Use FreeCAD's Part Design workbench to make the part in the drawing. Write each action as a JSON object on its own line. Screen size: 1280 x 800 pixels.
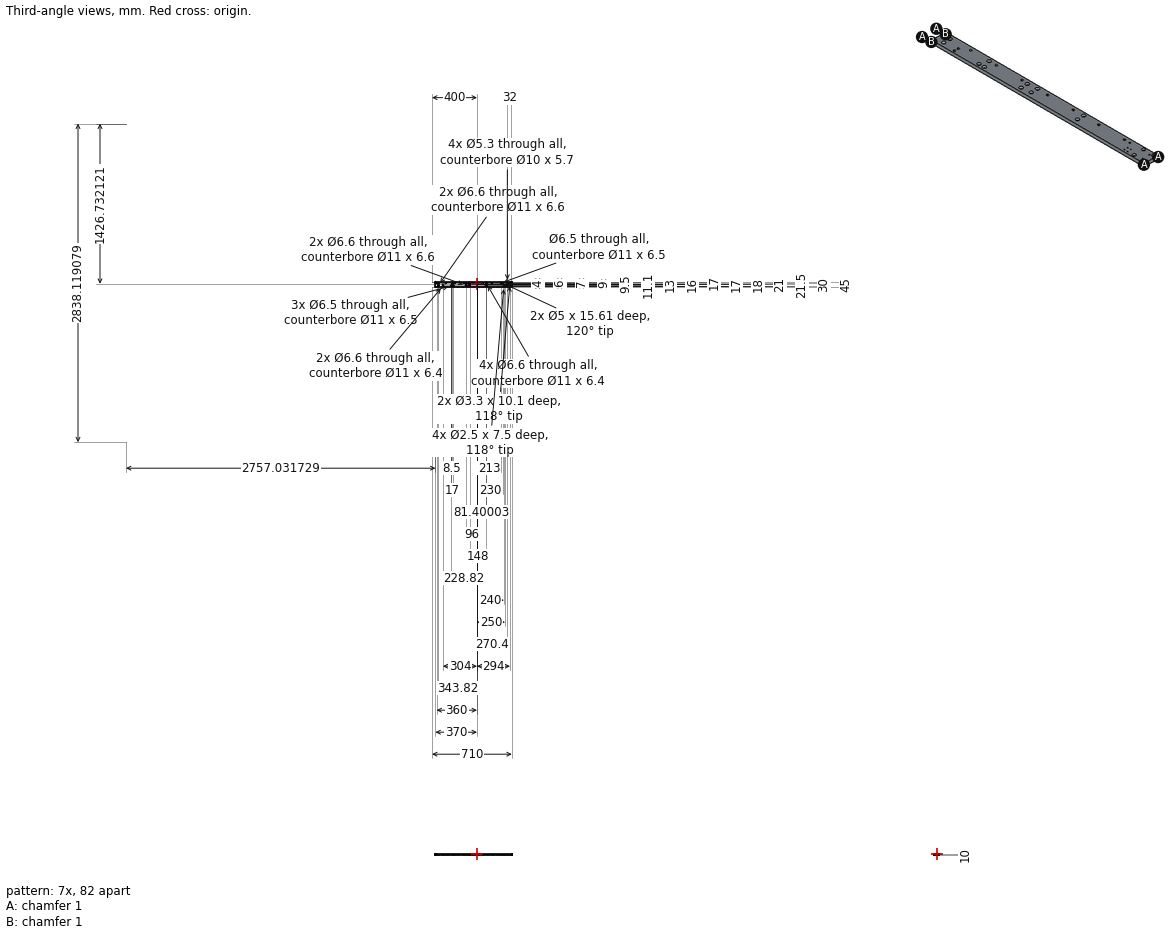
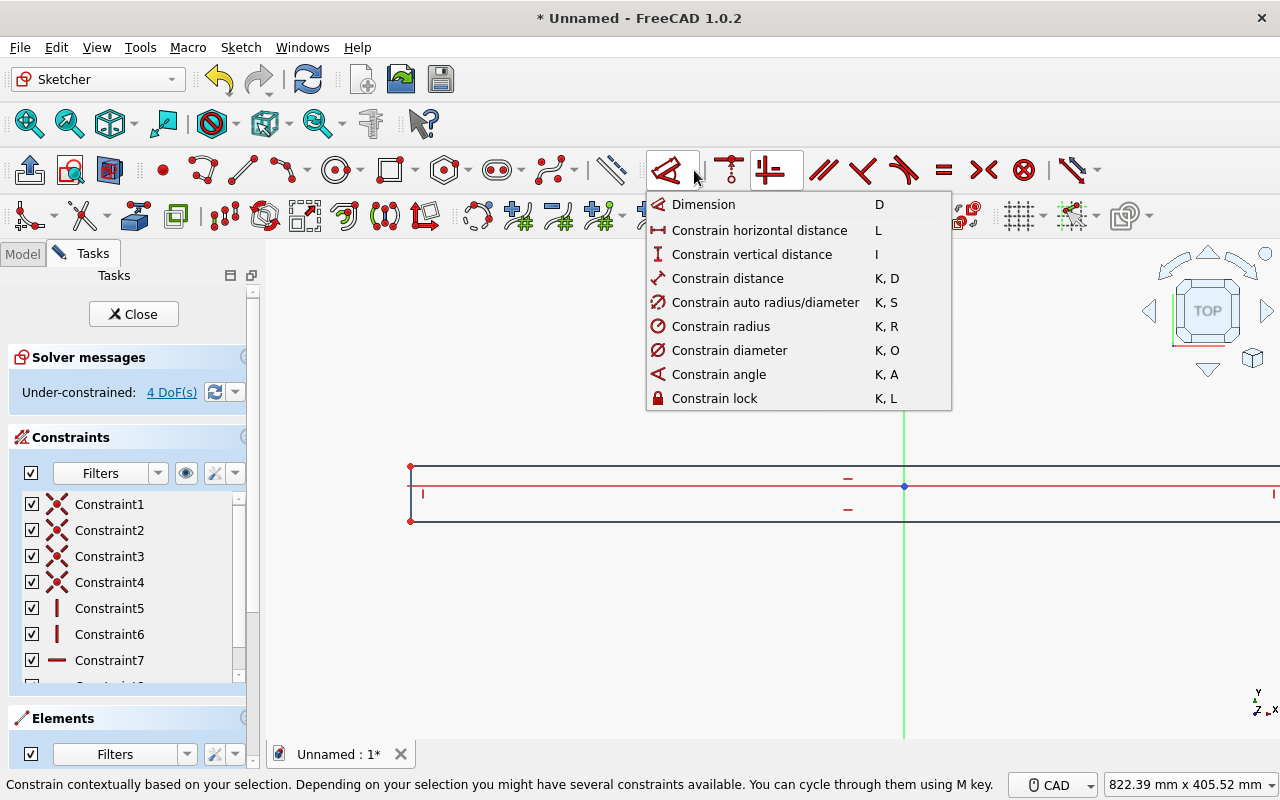
{"action": "left_click", "coordinate": [799, 254]}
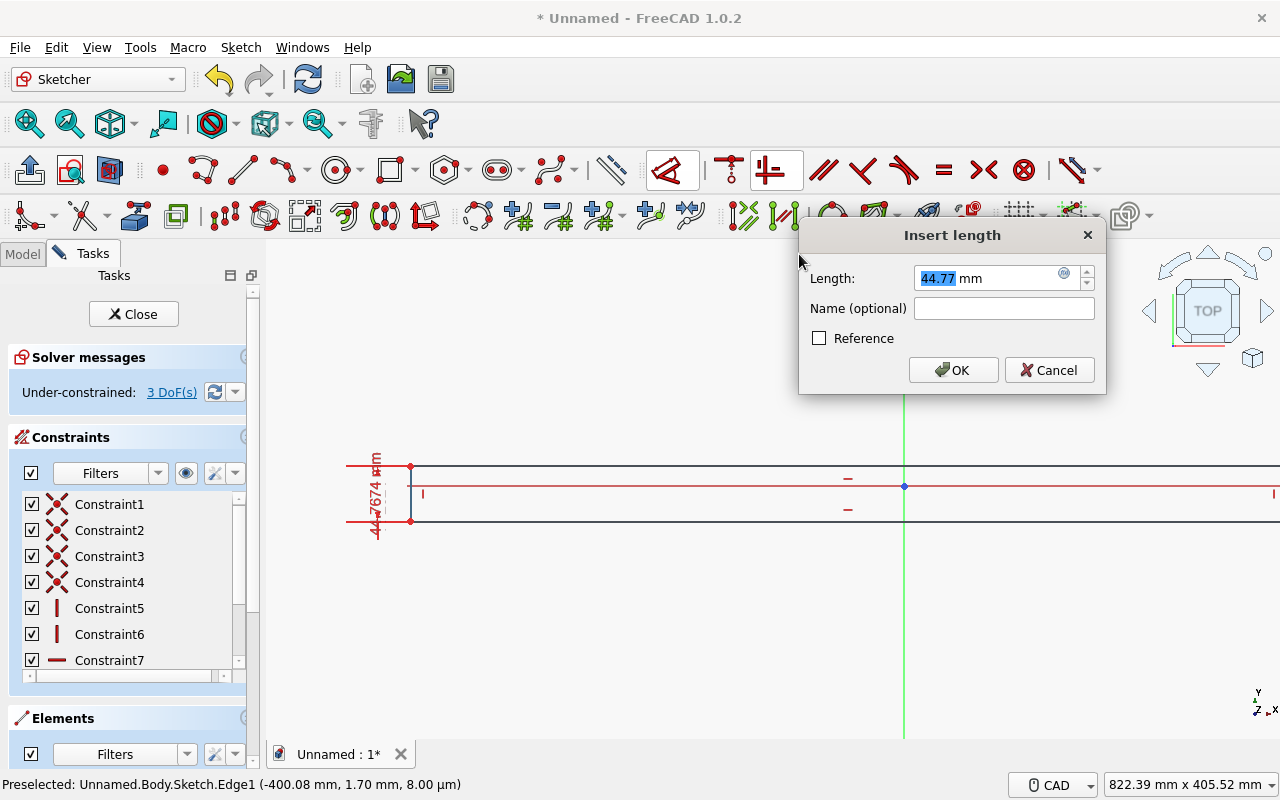
{"action": "type", "text": "45"}
{"action": "key", "text": "Return"}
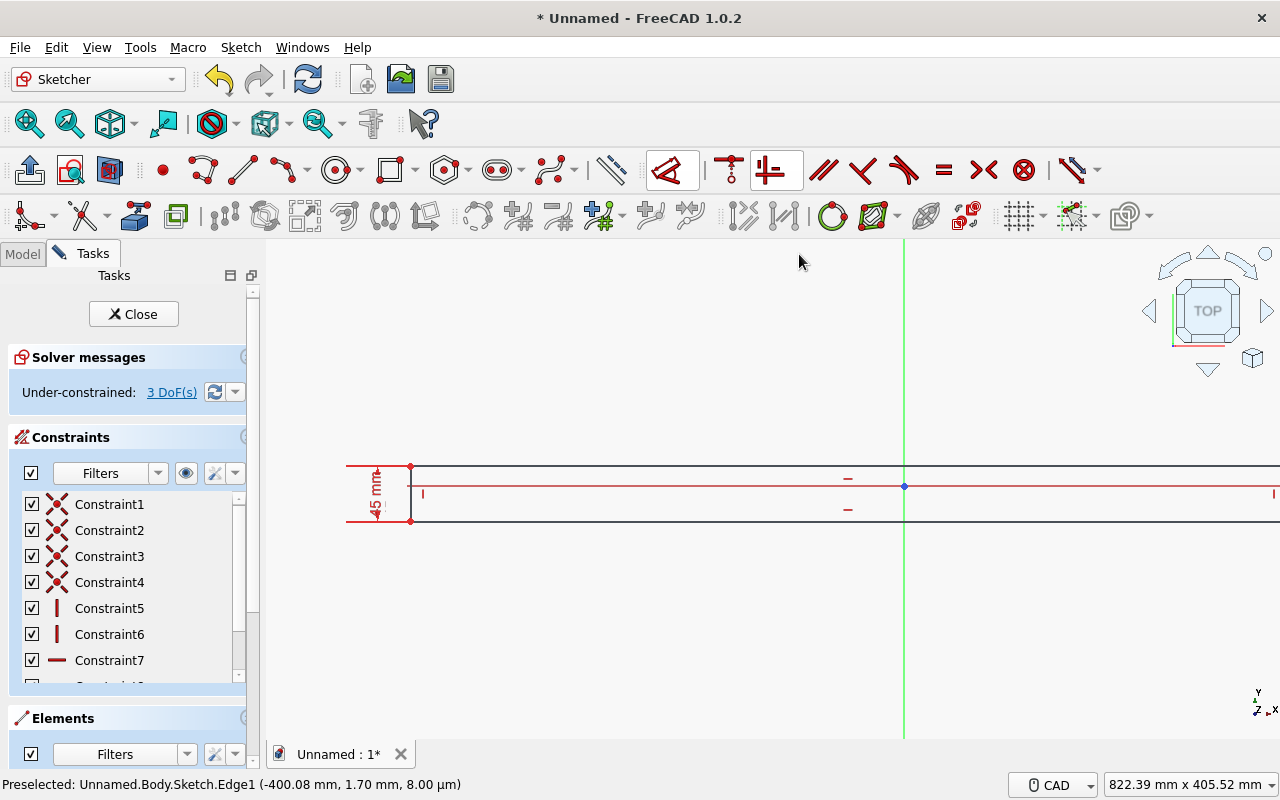
{"action": "left_click", "coordinate": [674, 522]}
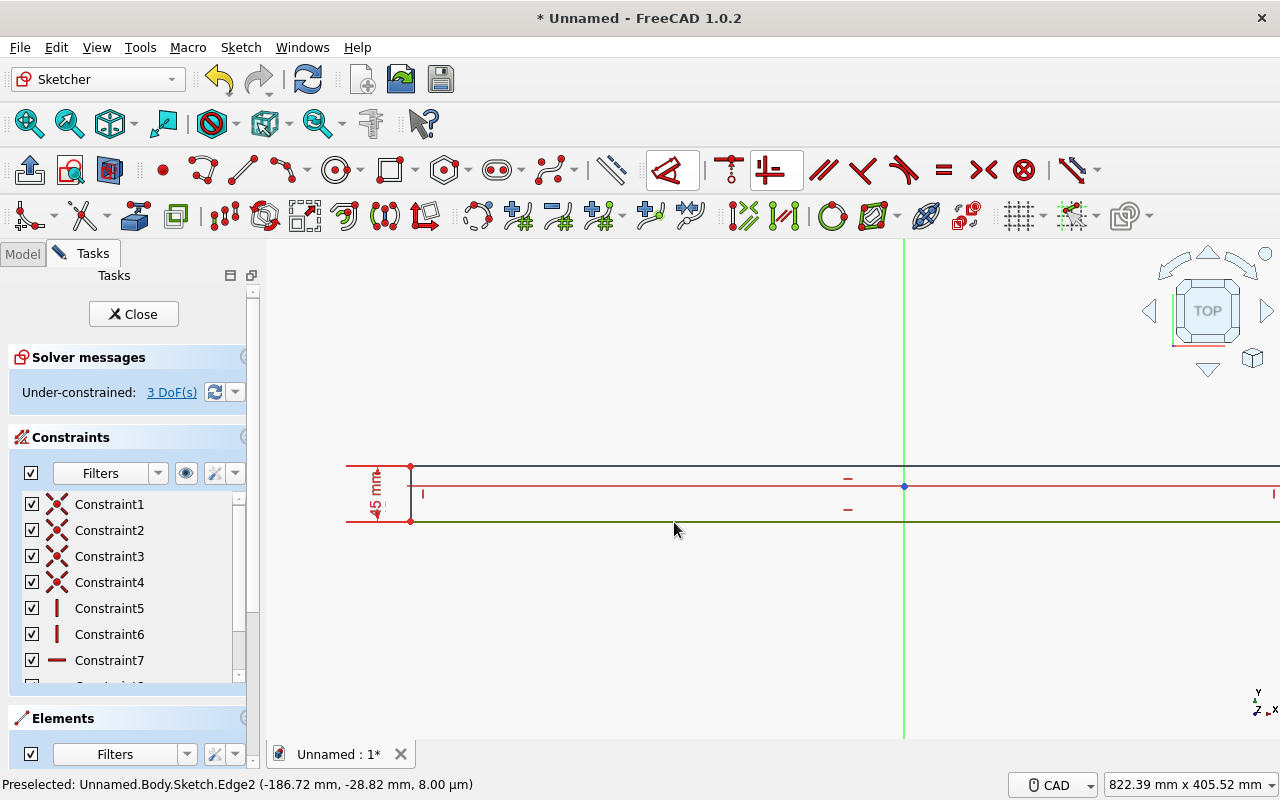
{"action": "key", "text": "l"}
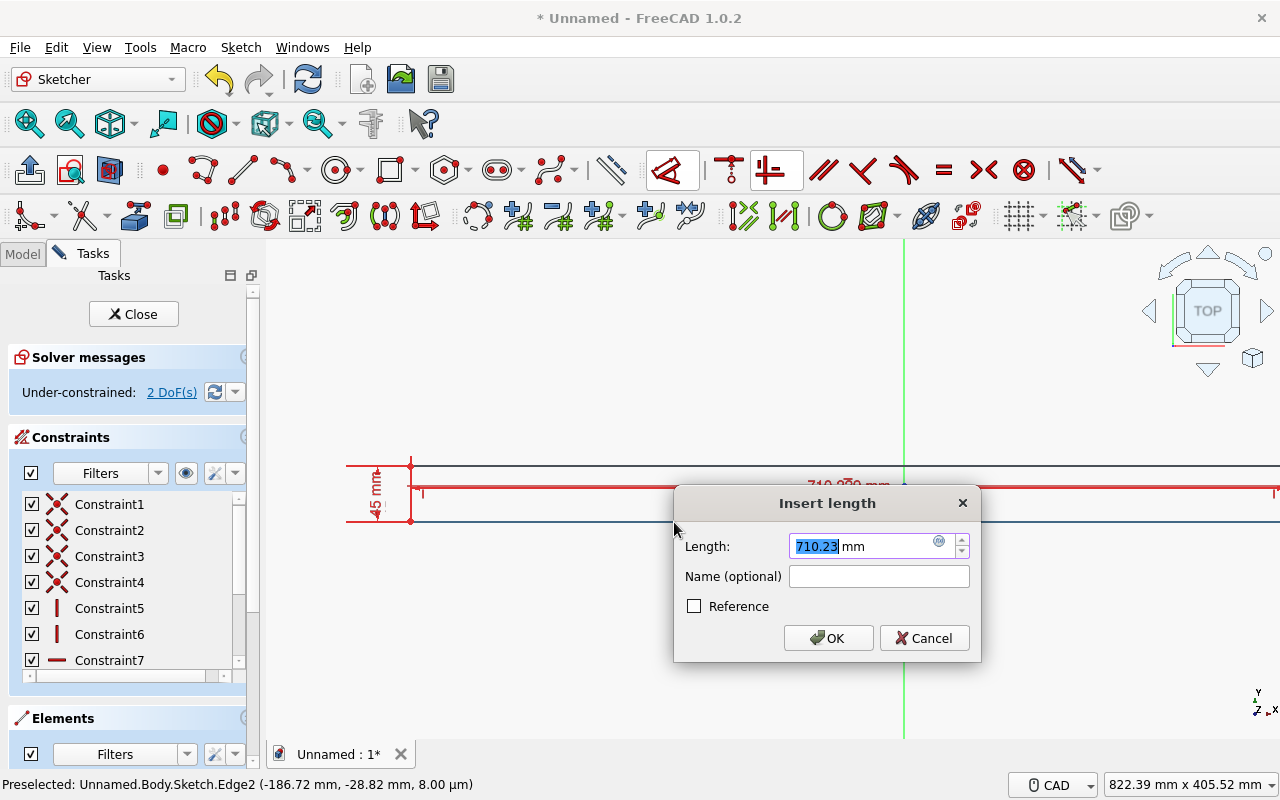
{"action": "type", "text": "710"}
{"action": "key", "text": "Return"}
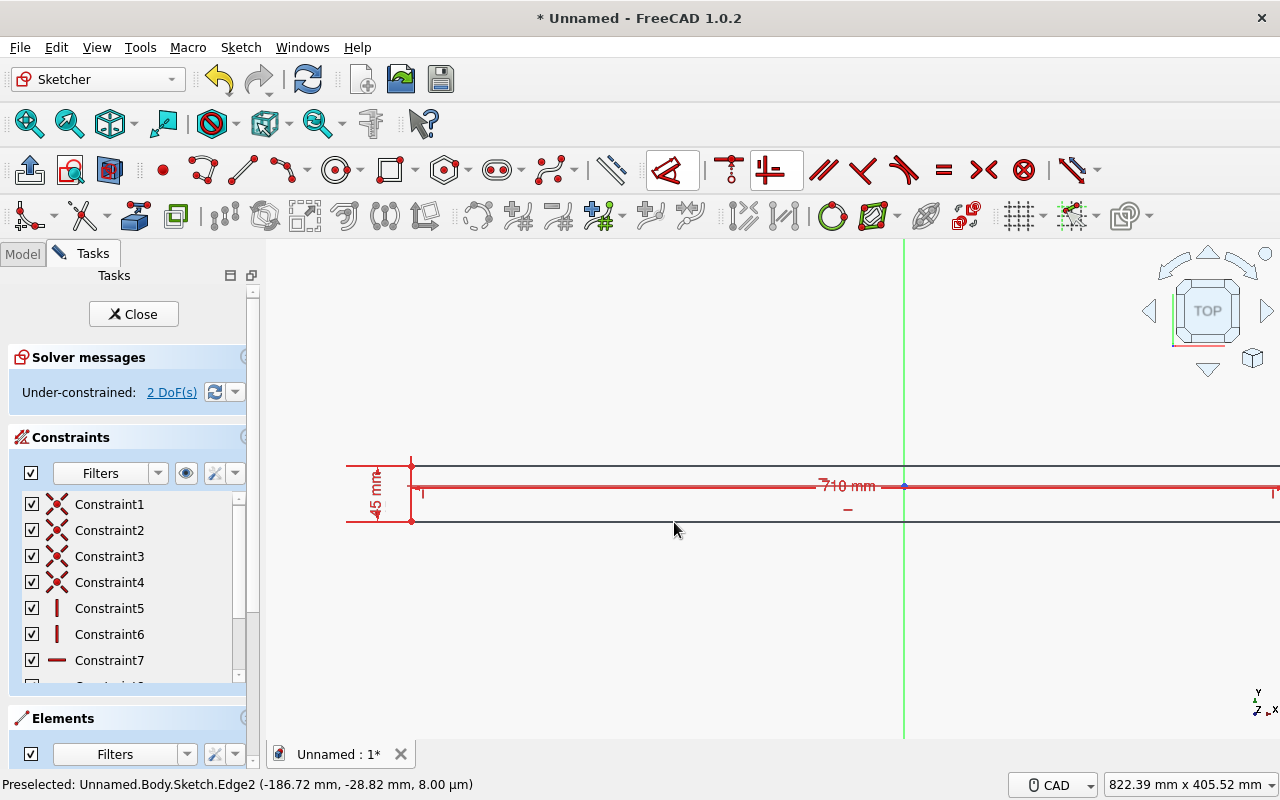
{"action": "scroll", "coordinate": [411, 466], "scroll_direction": "up", "scroll_amount": 4}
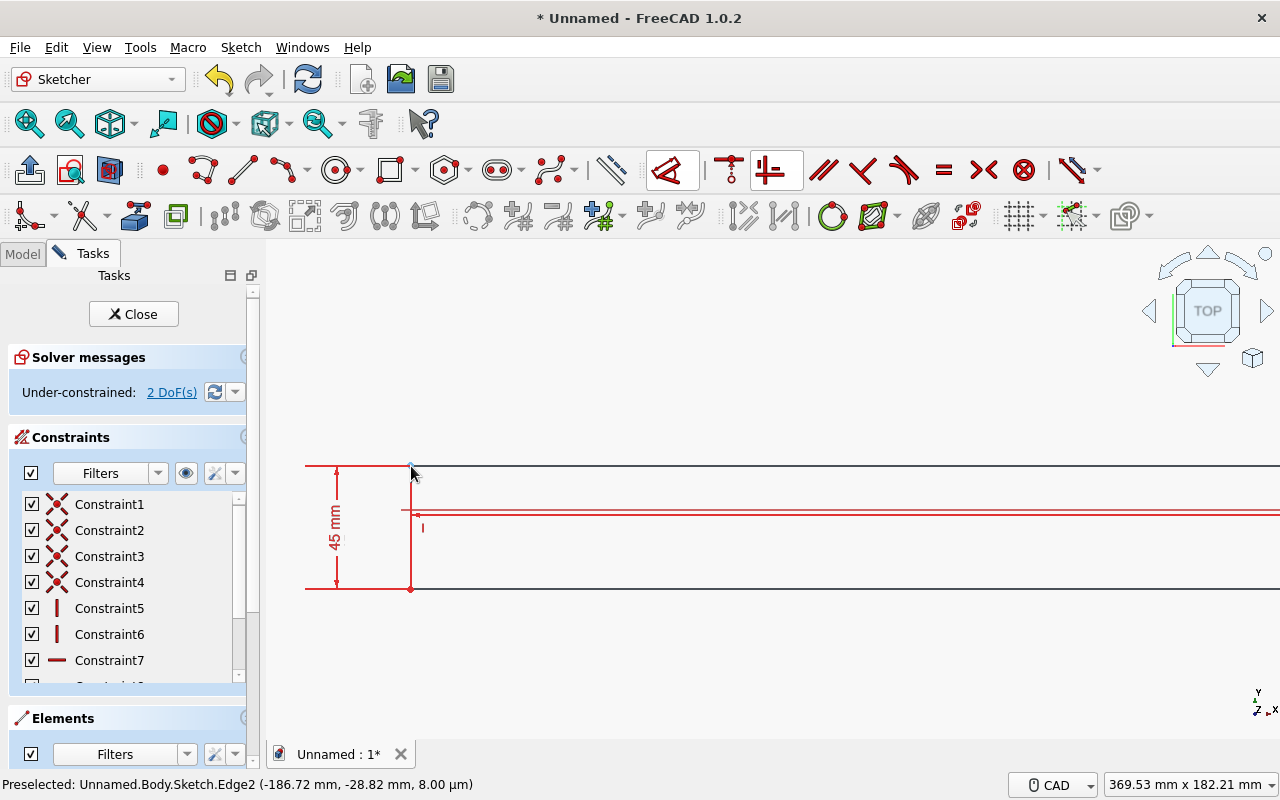
{"action": "left_click", "coordinate": [411, 466]}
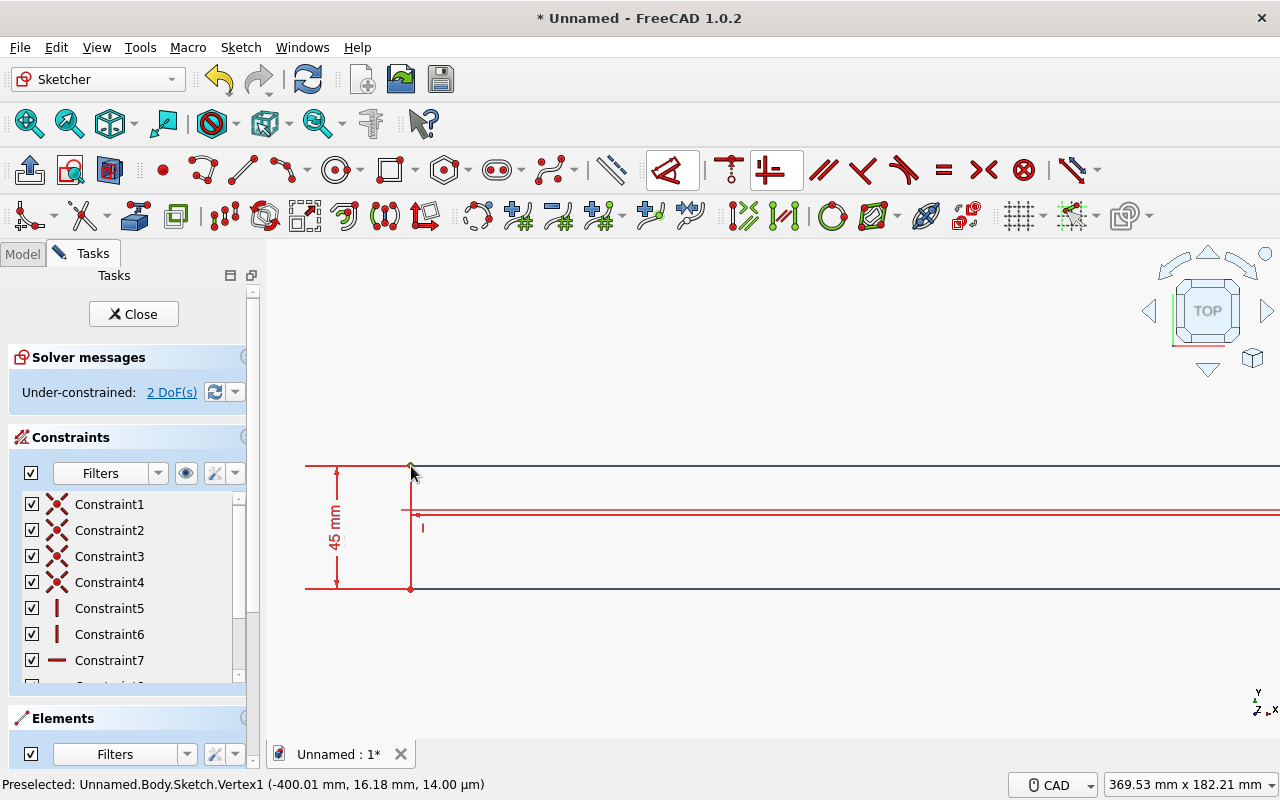
{"action": "key", "text": "i"}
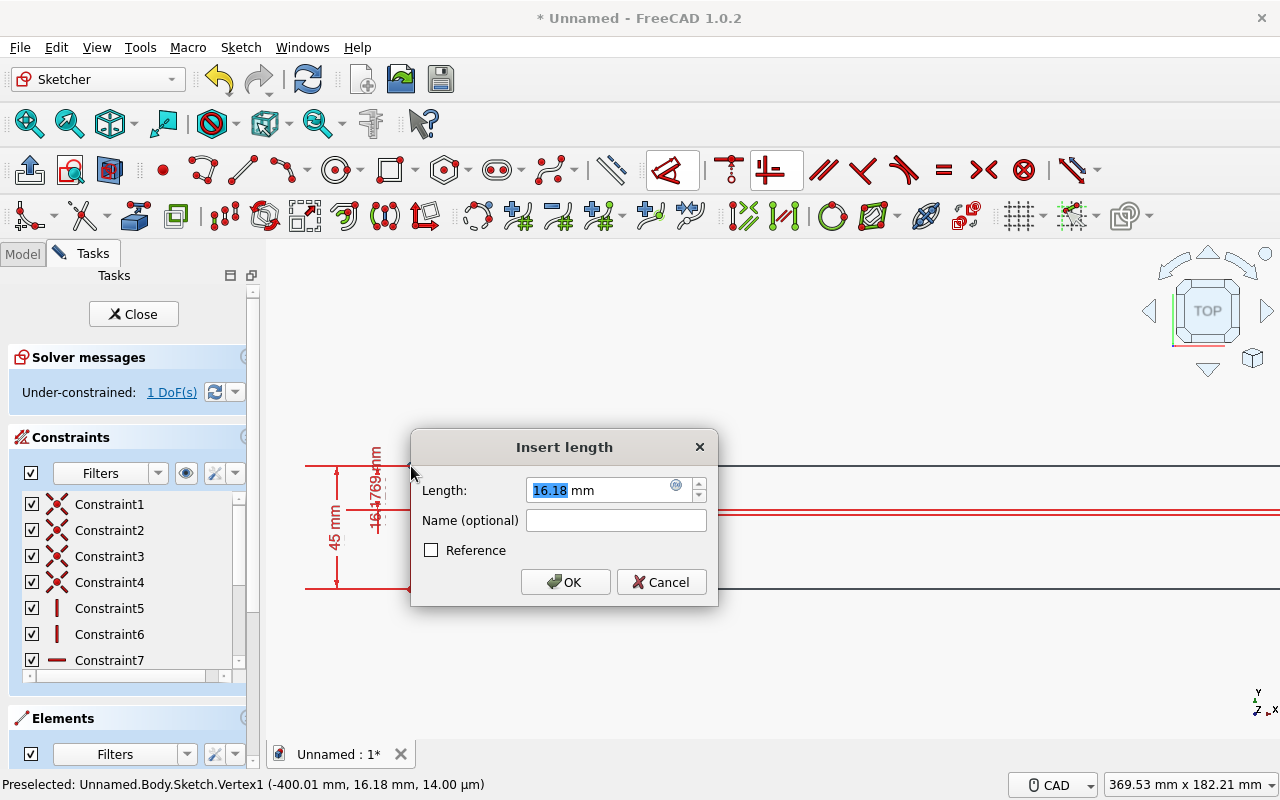
{"action": "type", "text": "17"}
{"action": "key", "text": "Return"}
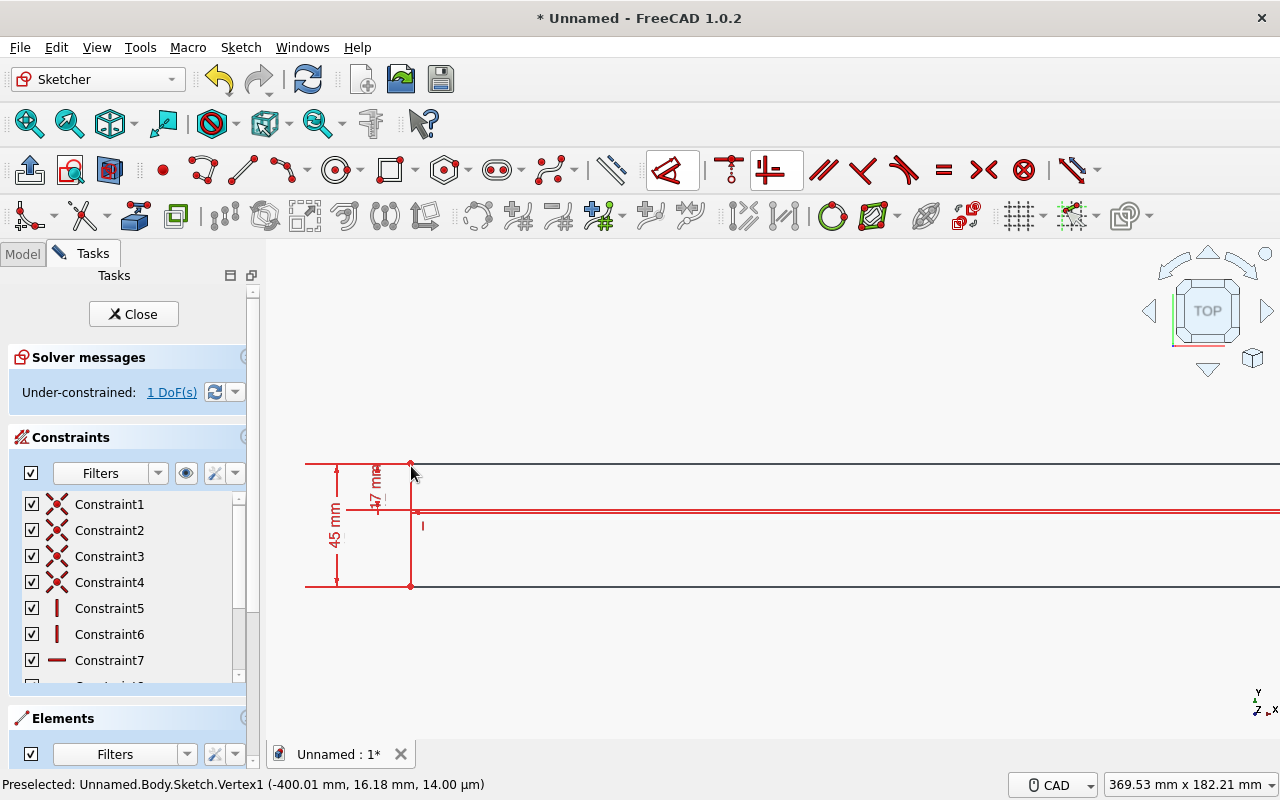
{"action": "left_click", "coordinate": [411, 464]}